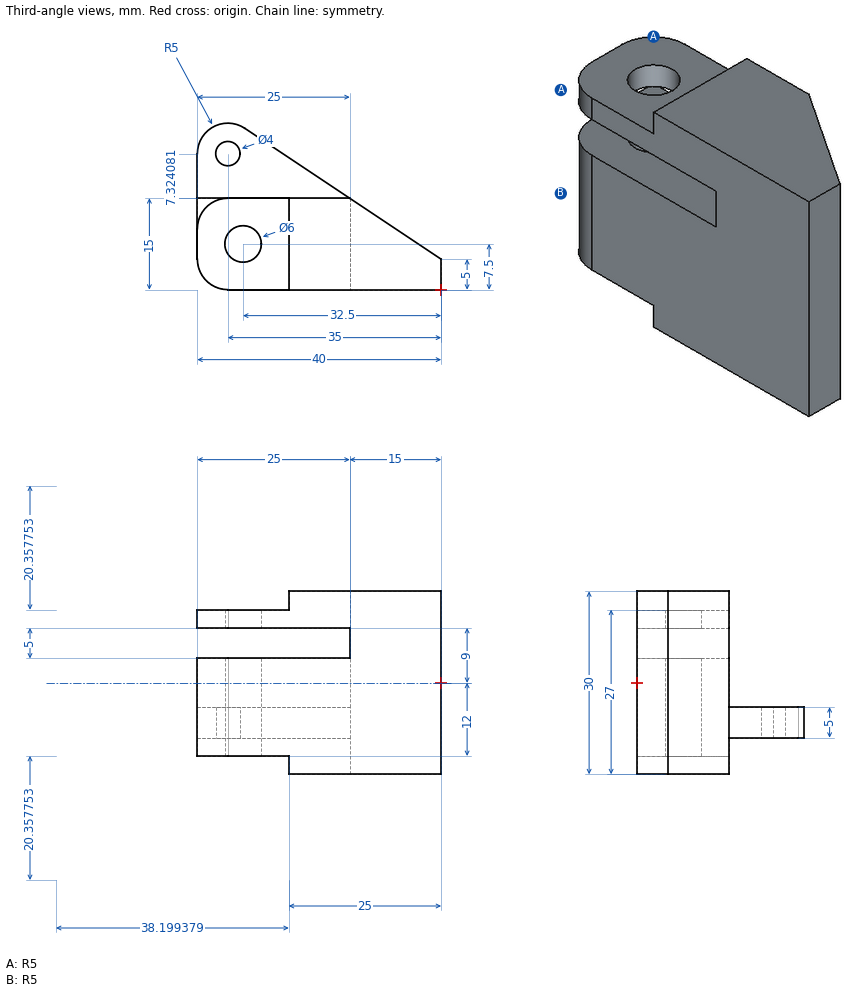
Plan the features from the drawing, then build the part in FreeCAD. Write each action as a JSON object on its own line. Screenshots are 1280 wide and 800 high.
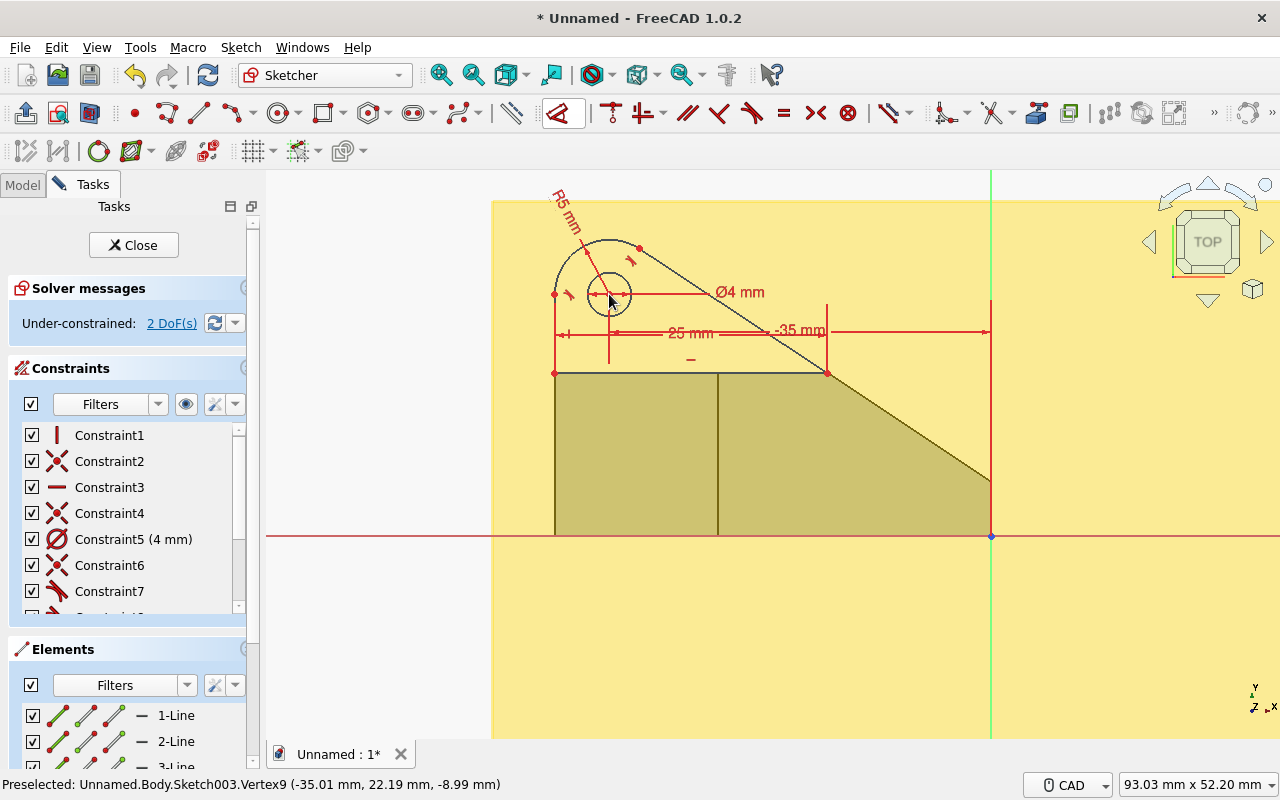
{"action": "left_click", "coordinate": [555, 373]}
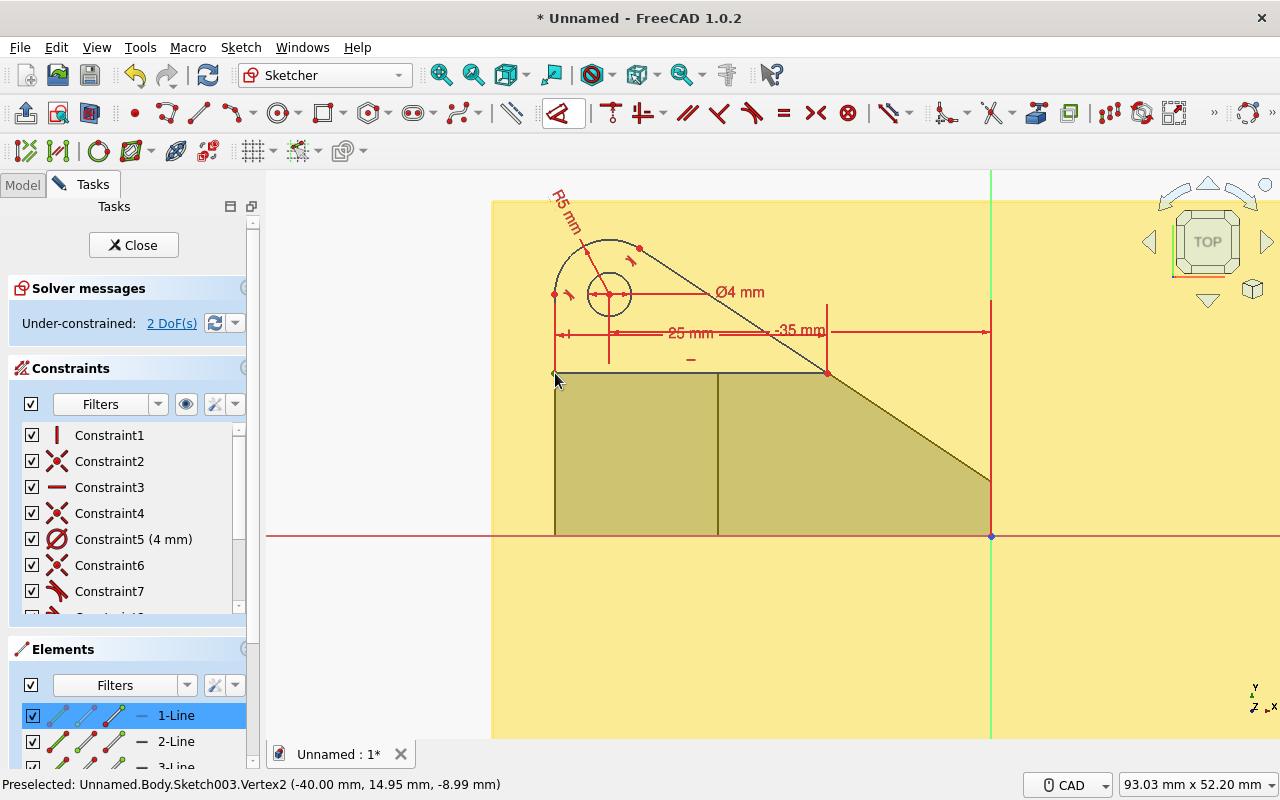
{"action": "key", "text": "i"}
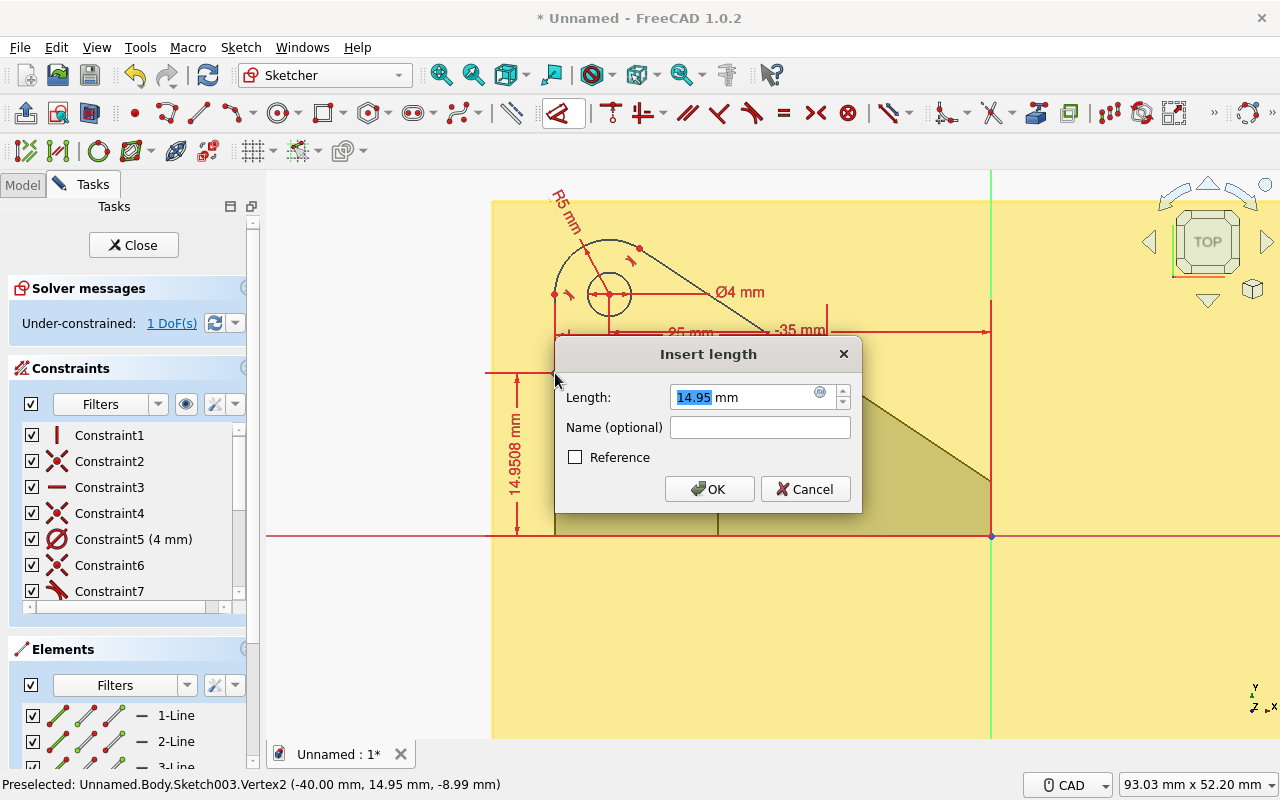
{"action": "type", "text": "15"}
{"action": "key", "text": "Return"}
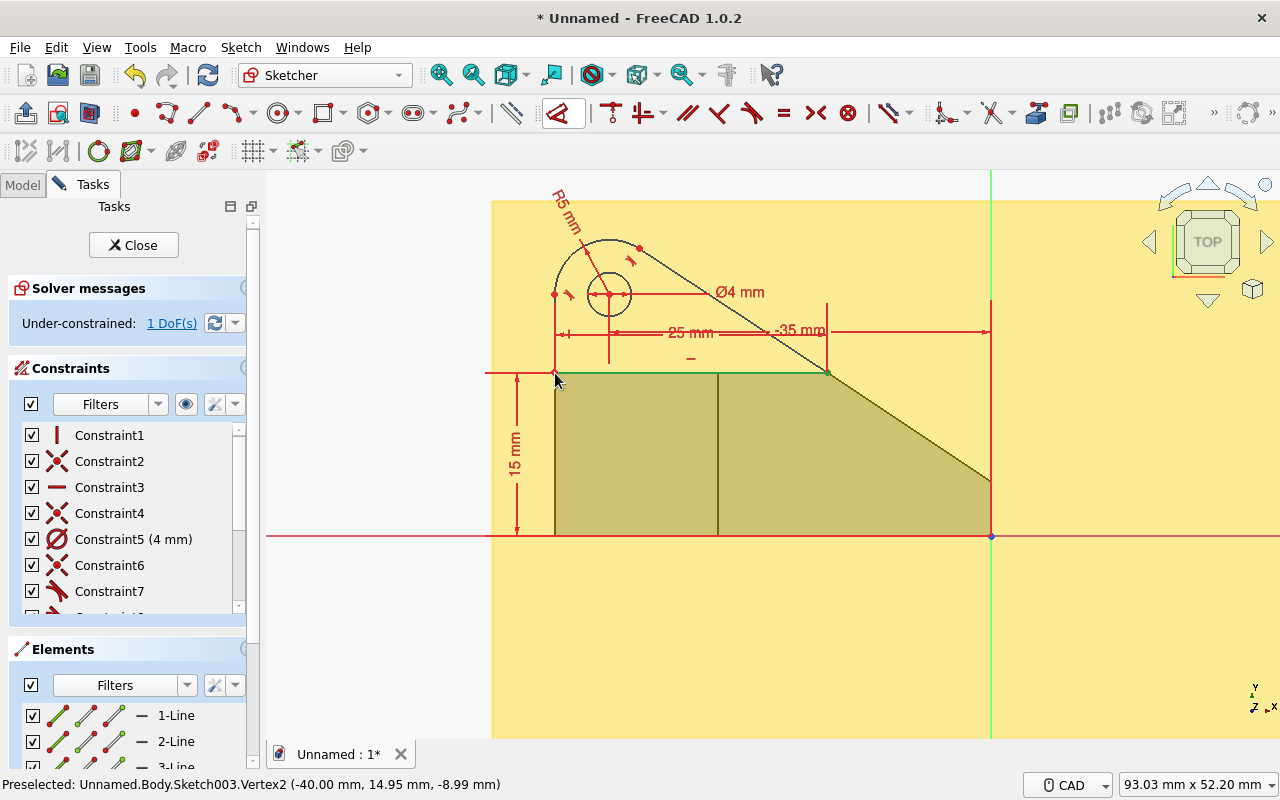
{"action": "left_click", "coordinate": [555, 318]}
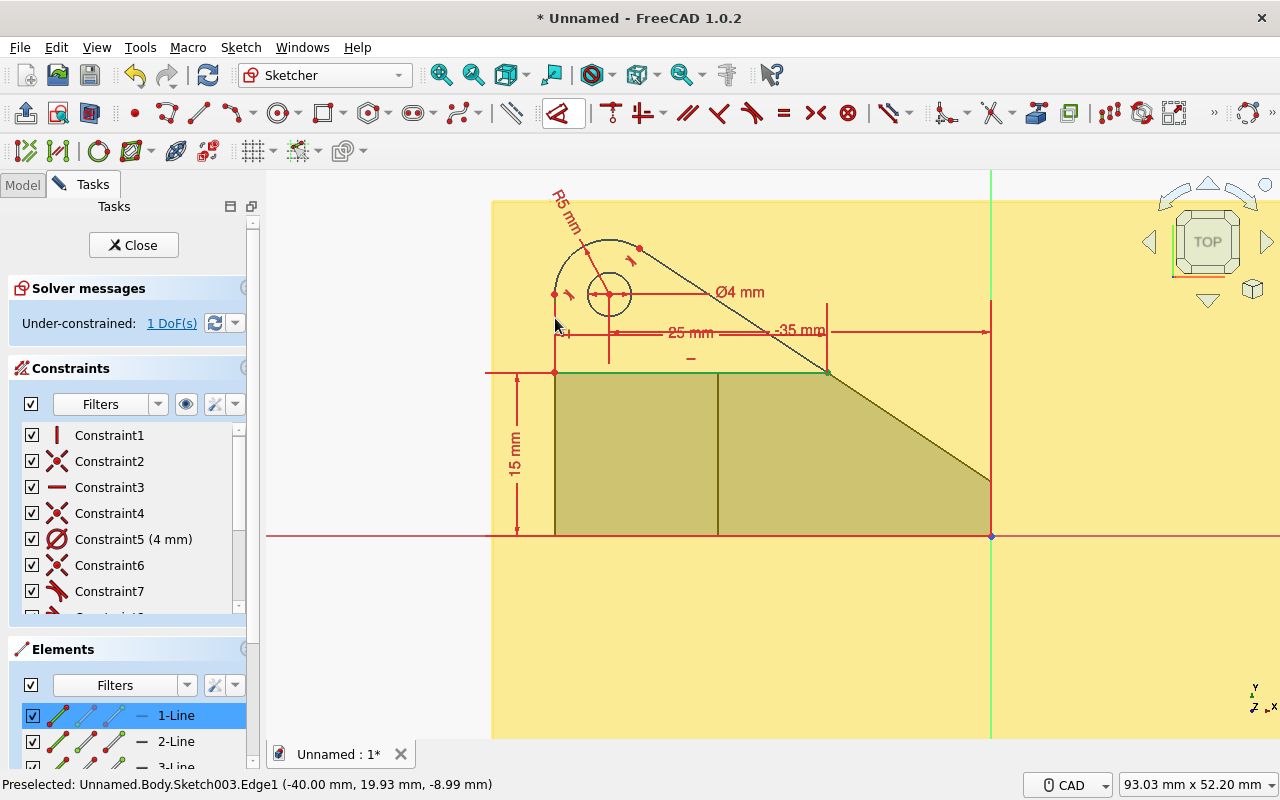
{"action": "key", "text": "i"}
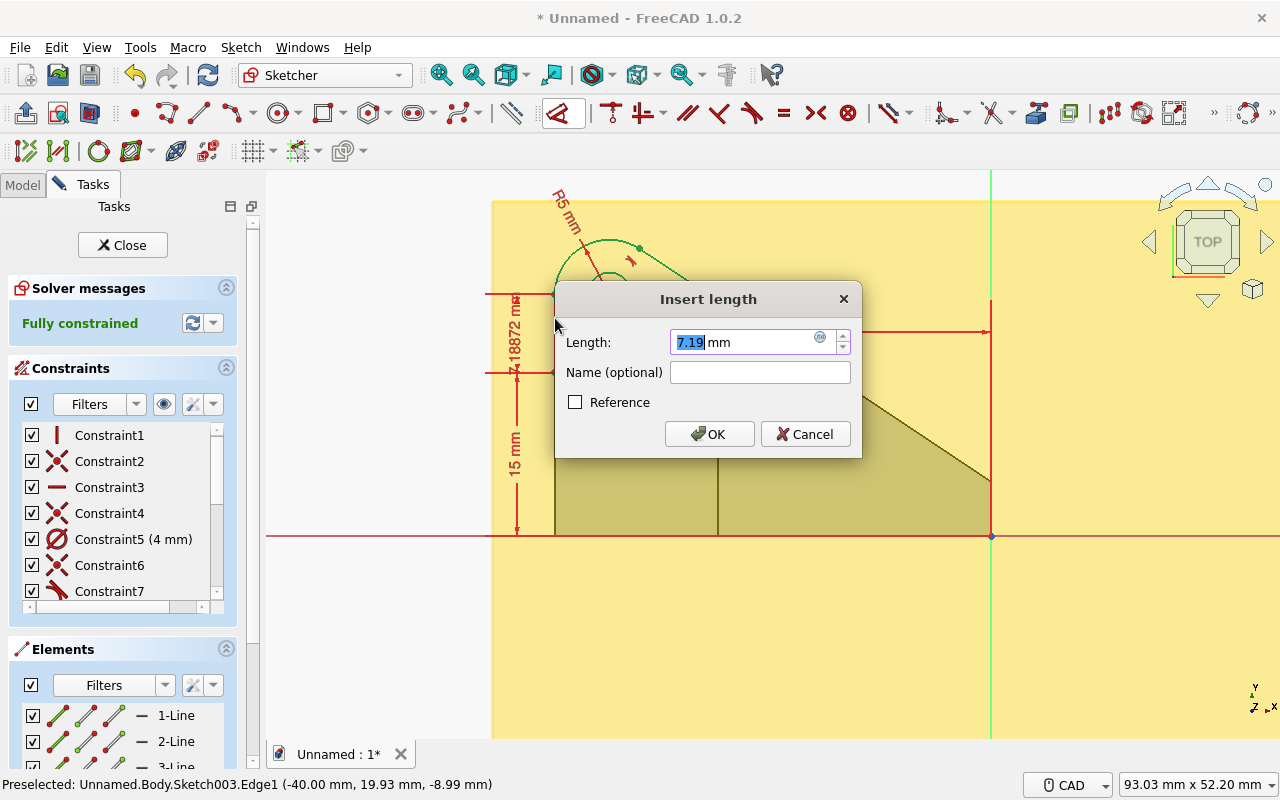
{"action": "type", "text": "7.324081"}
{"action": "key", "text": "Return"}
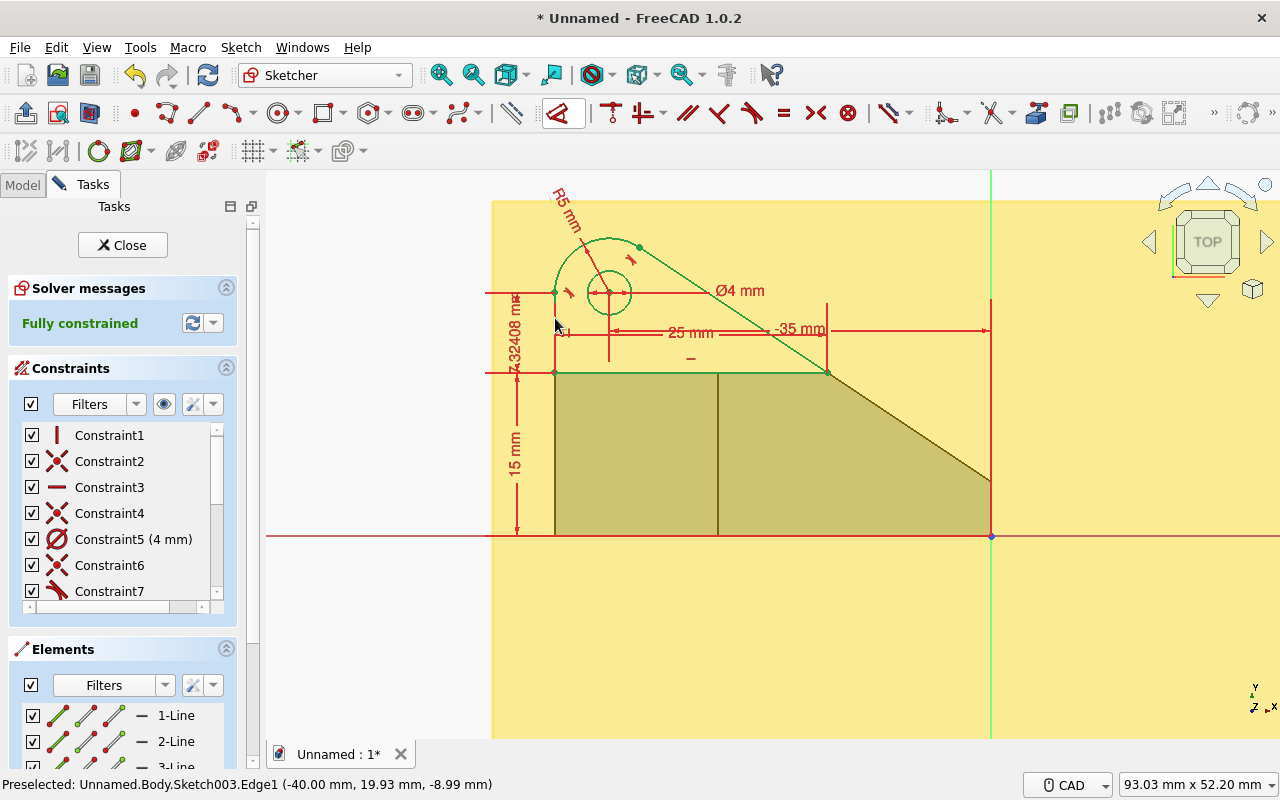
{"action": "left_click", "coordinate": [123, 245]}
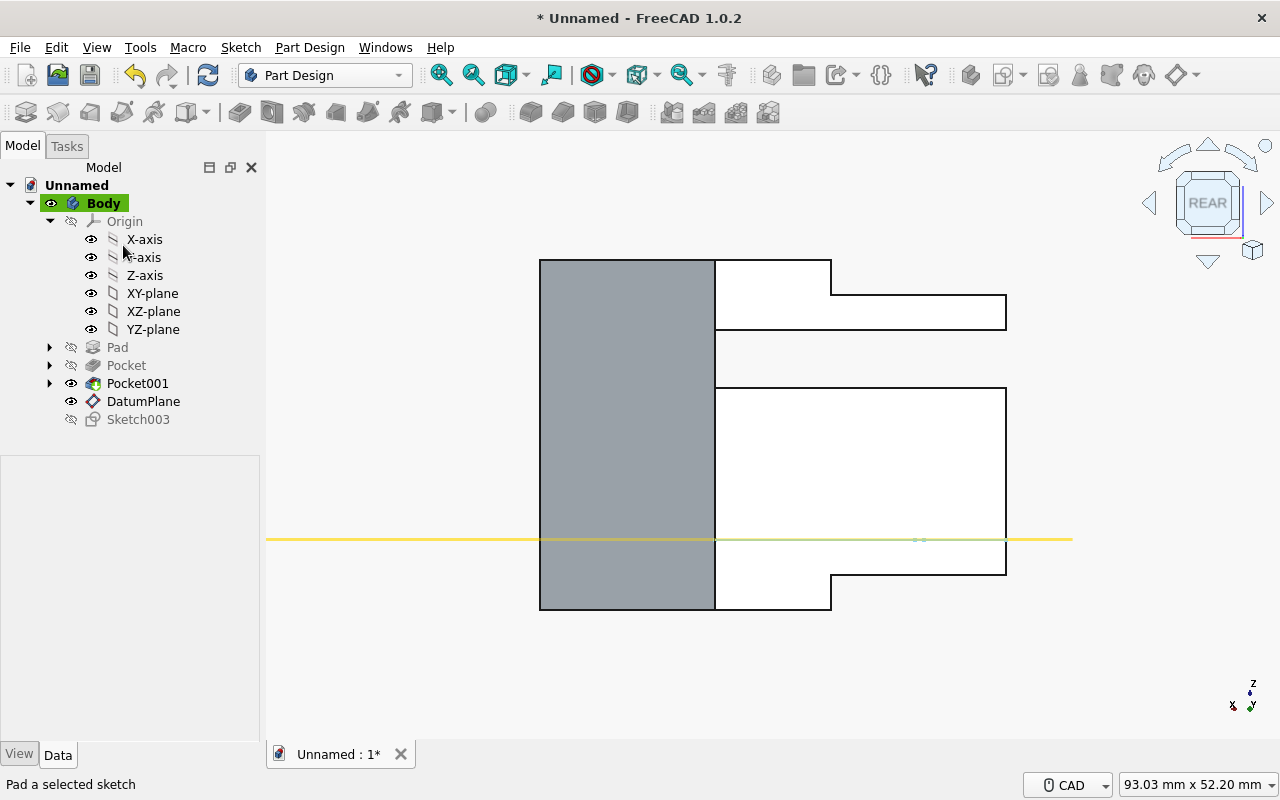
{"action": "left_click", "coordinate": [26, 112]}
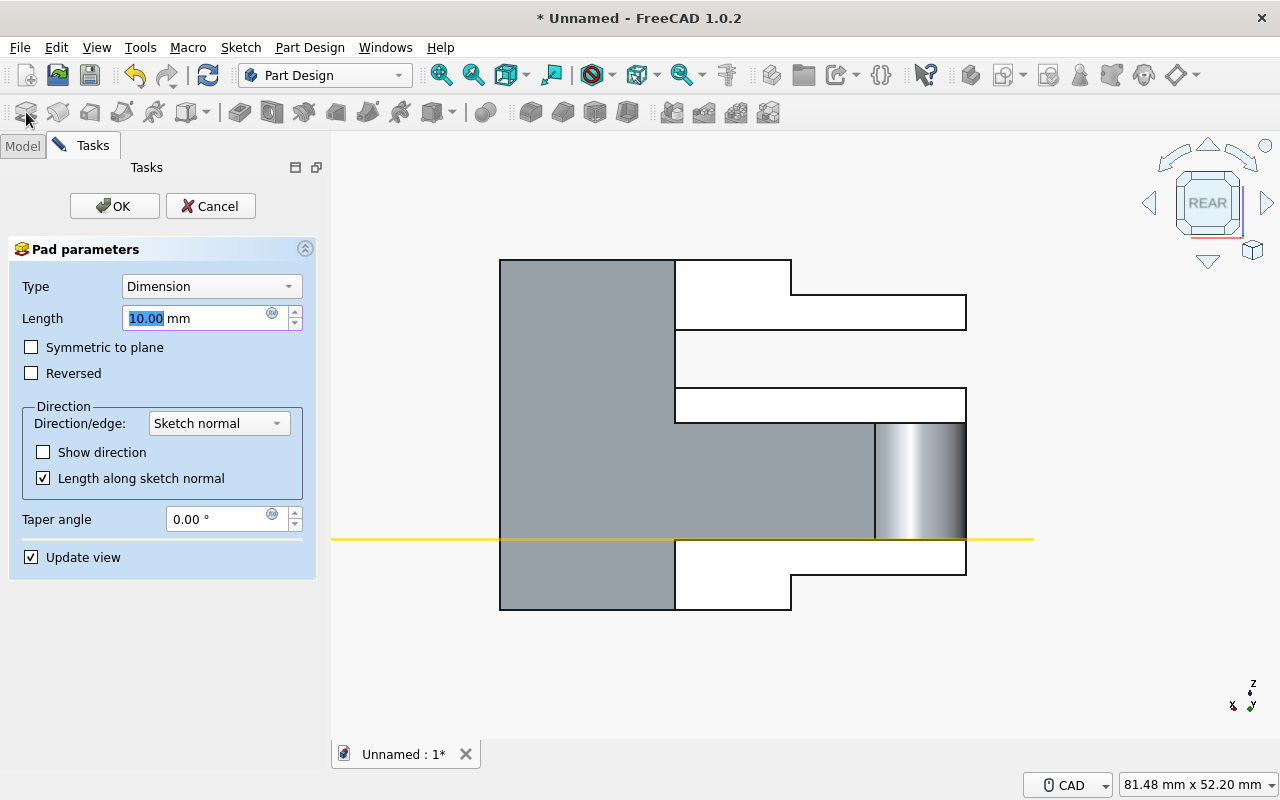
{"action": "type", "text": "5"}
{"action": "key", "text": "Tab"}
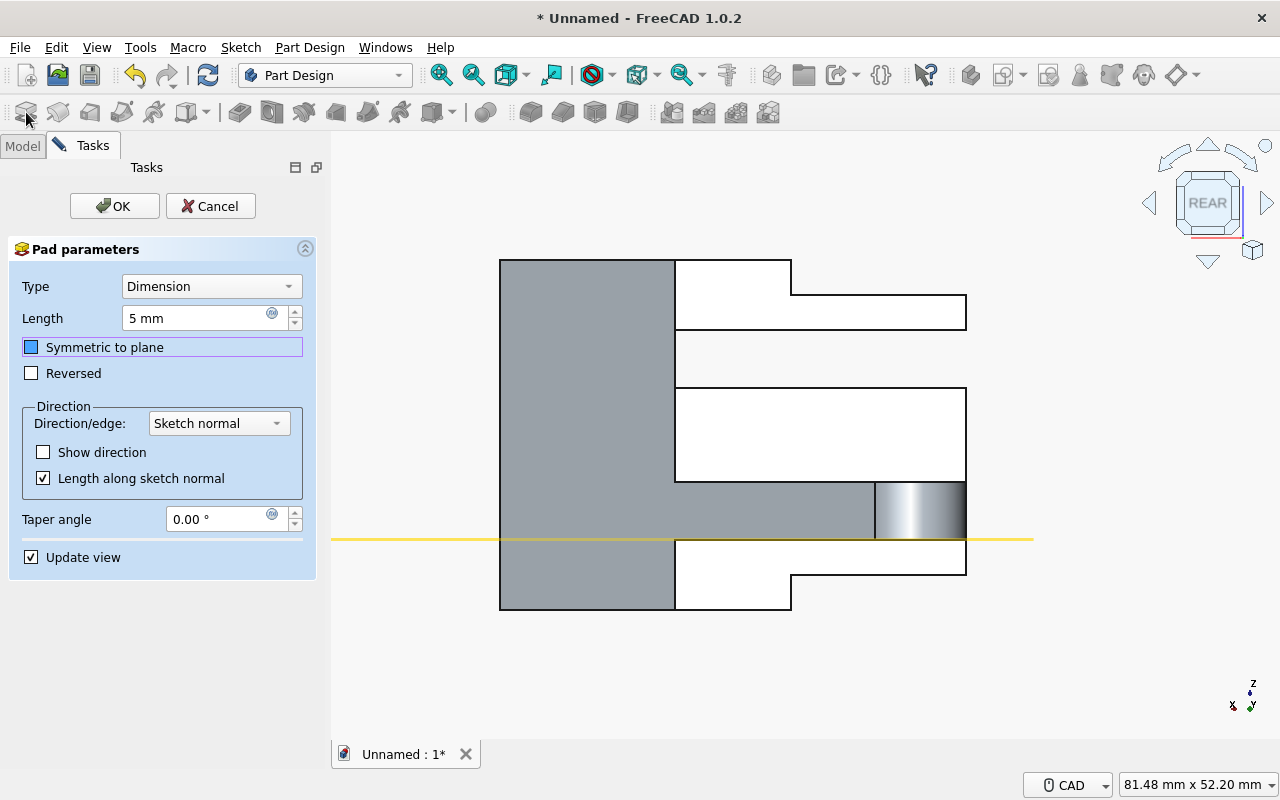
{"action": "left_click", "coordinate": [115, 206]}